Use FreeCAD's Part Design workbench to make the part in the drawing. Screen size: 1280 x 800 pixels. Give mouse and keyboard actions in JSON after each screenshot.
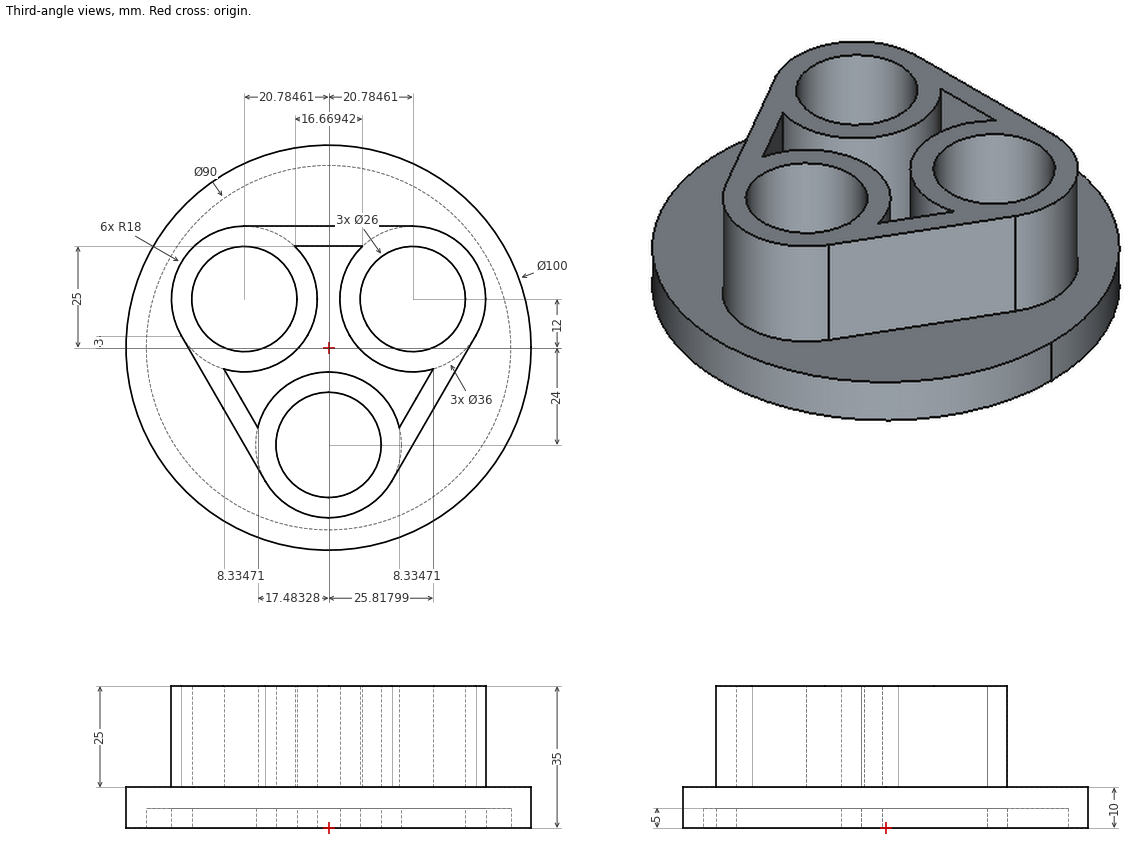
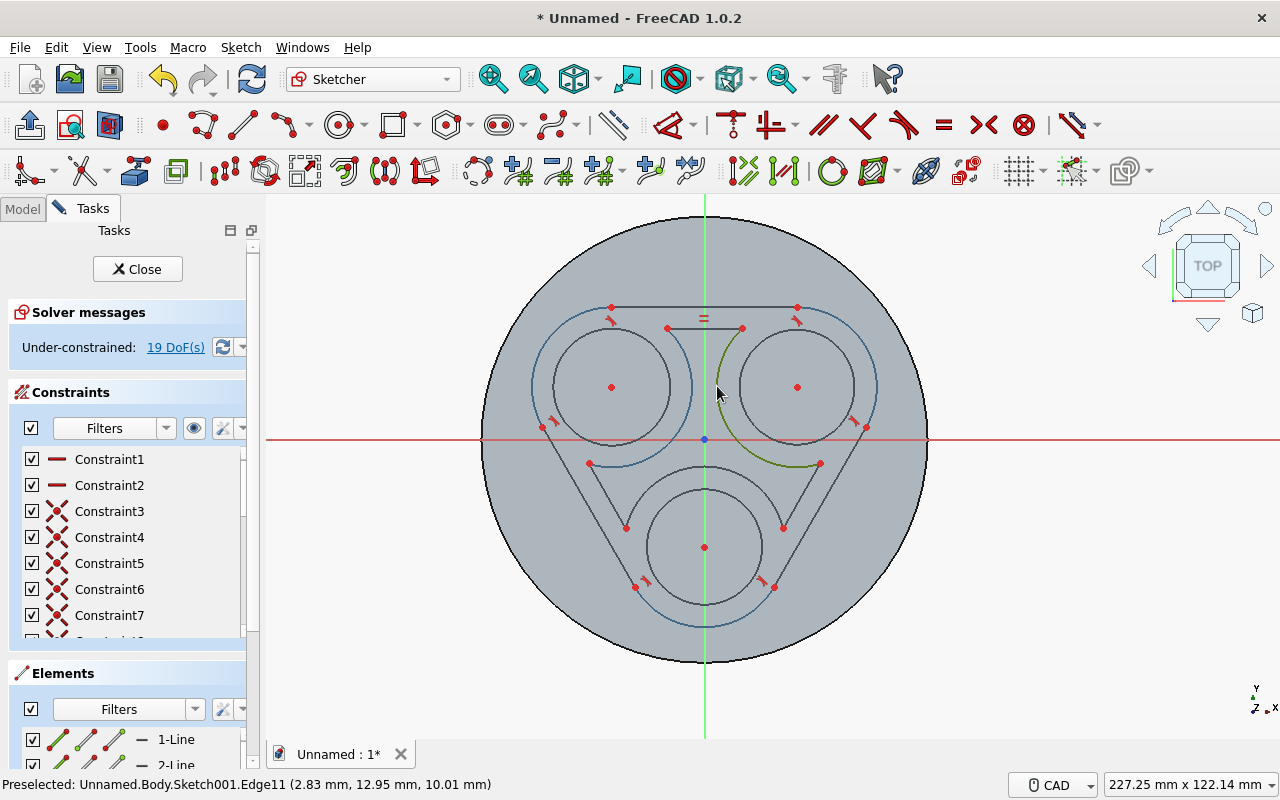
{"action": "left_click", "coordinate": [746, 478]}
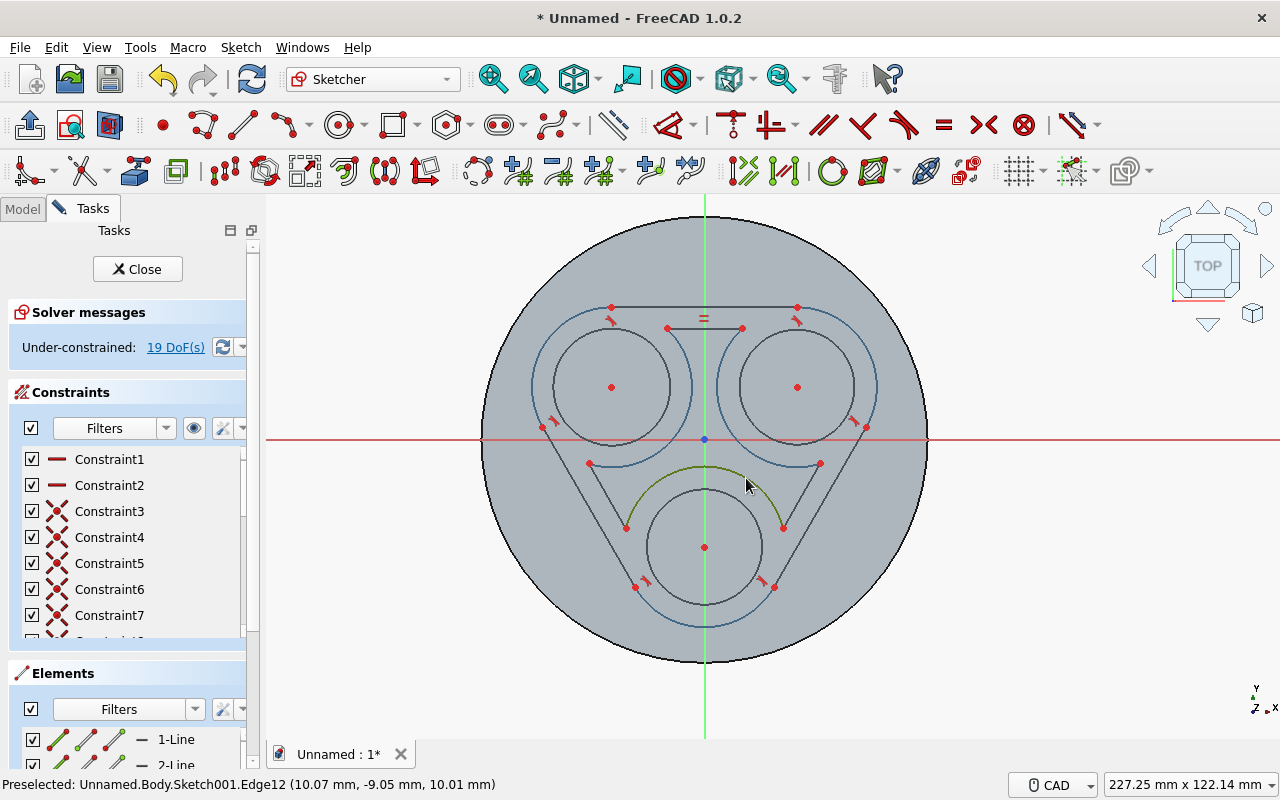
{"action": "left_click", "coordinate": [944, 126]}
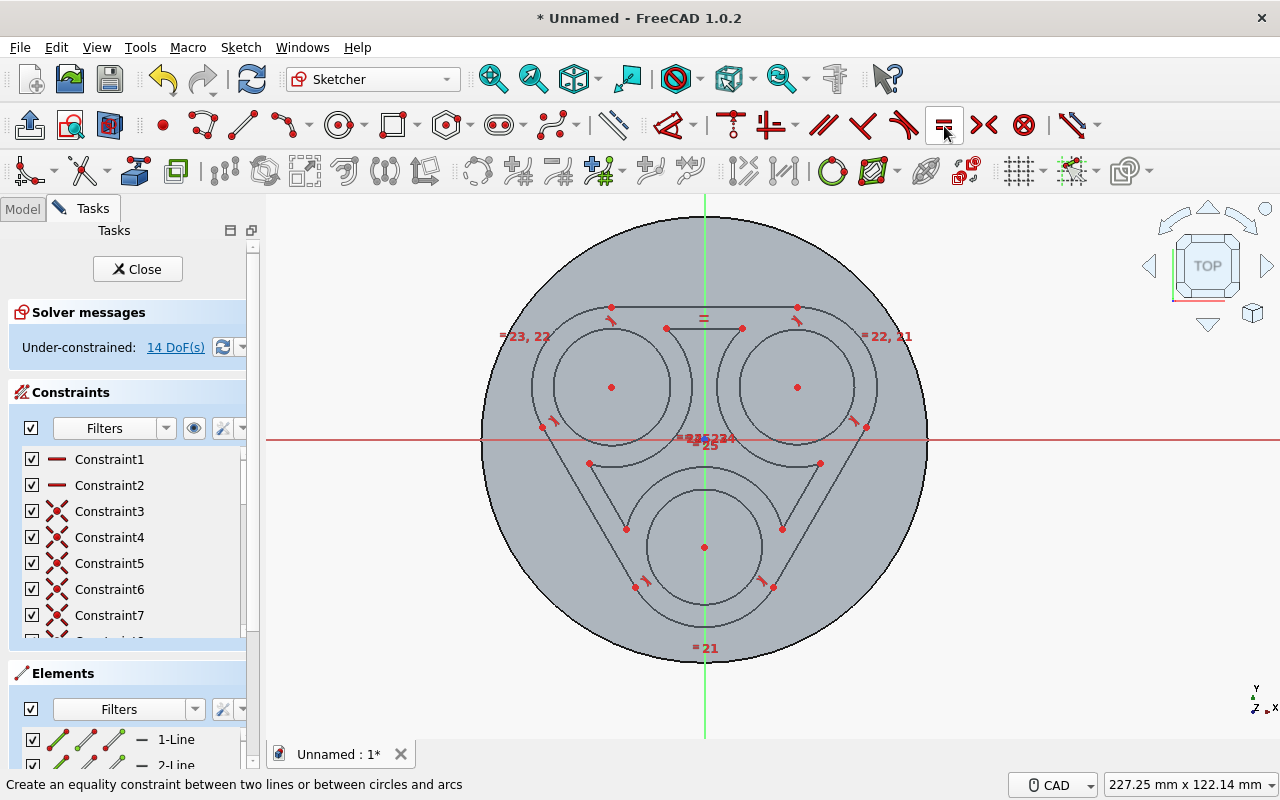
{"action": "left_click", "coordinate": [838, 346]}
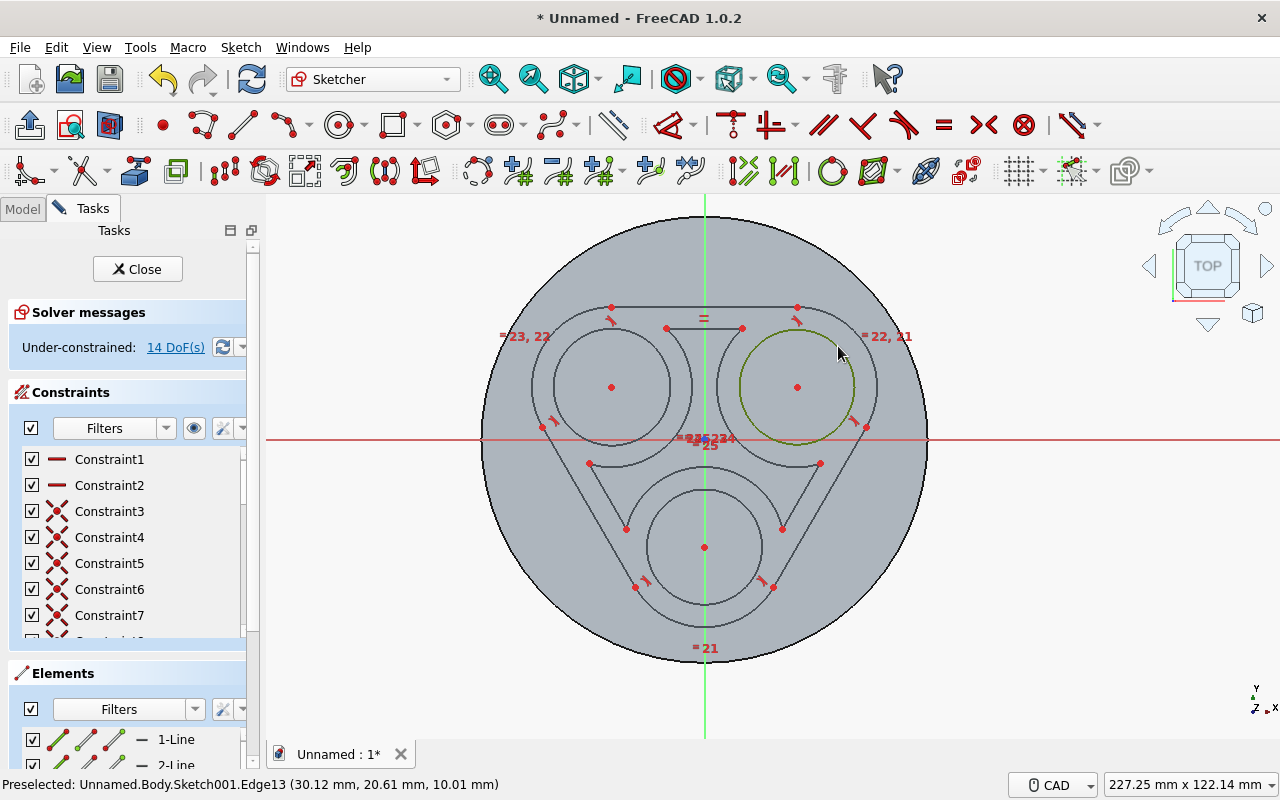
{"action": "left_click", "coordinate": [745, 506]}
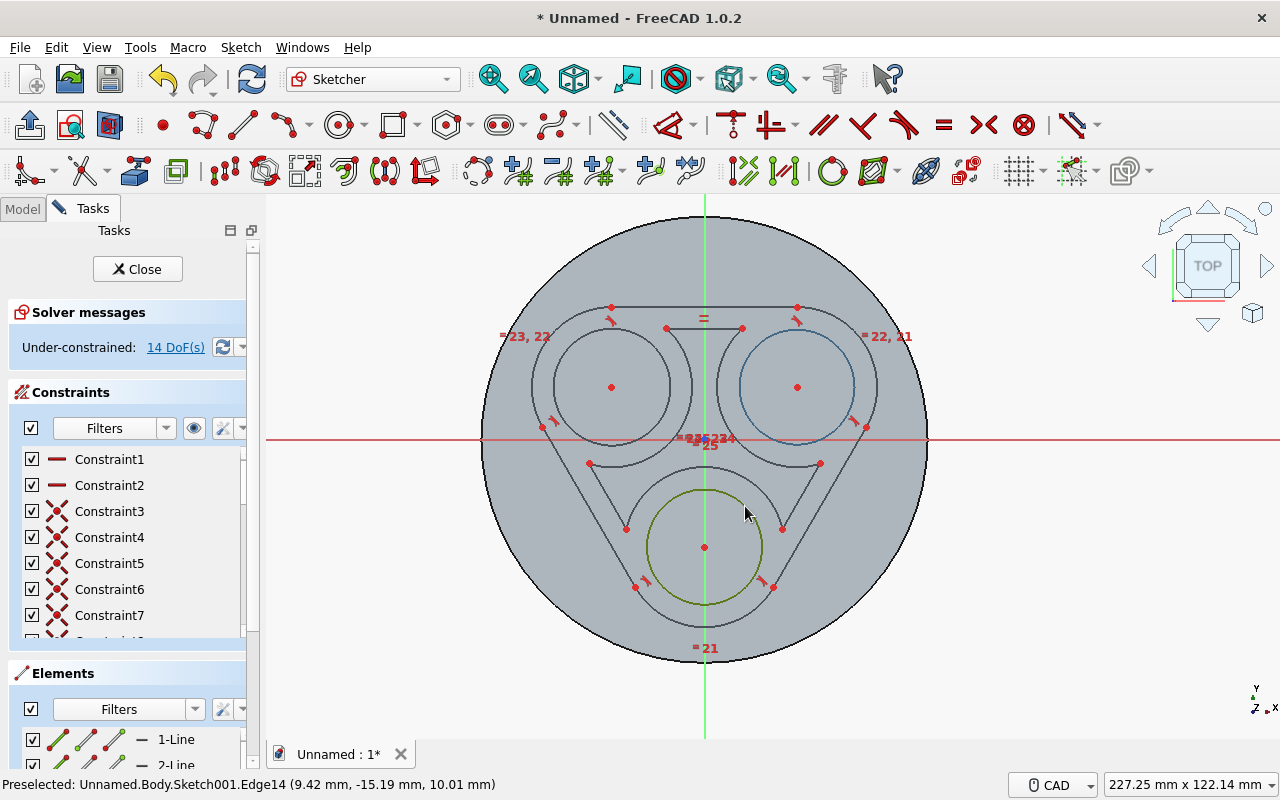
{"action": "left_click", "coordinate": [653, 346]}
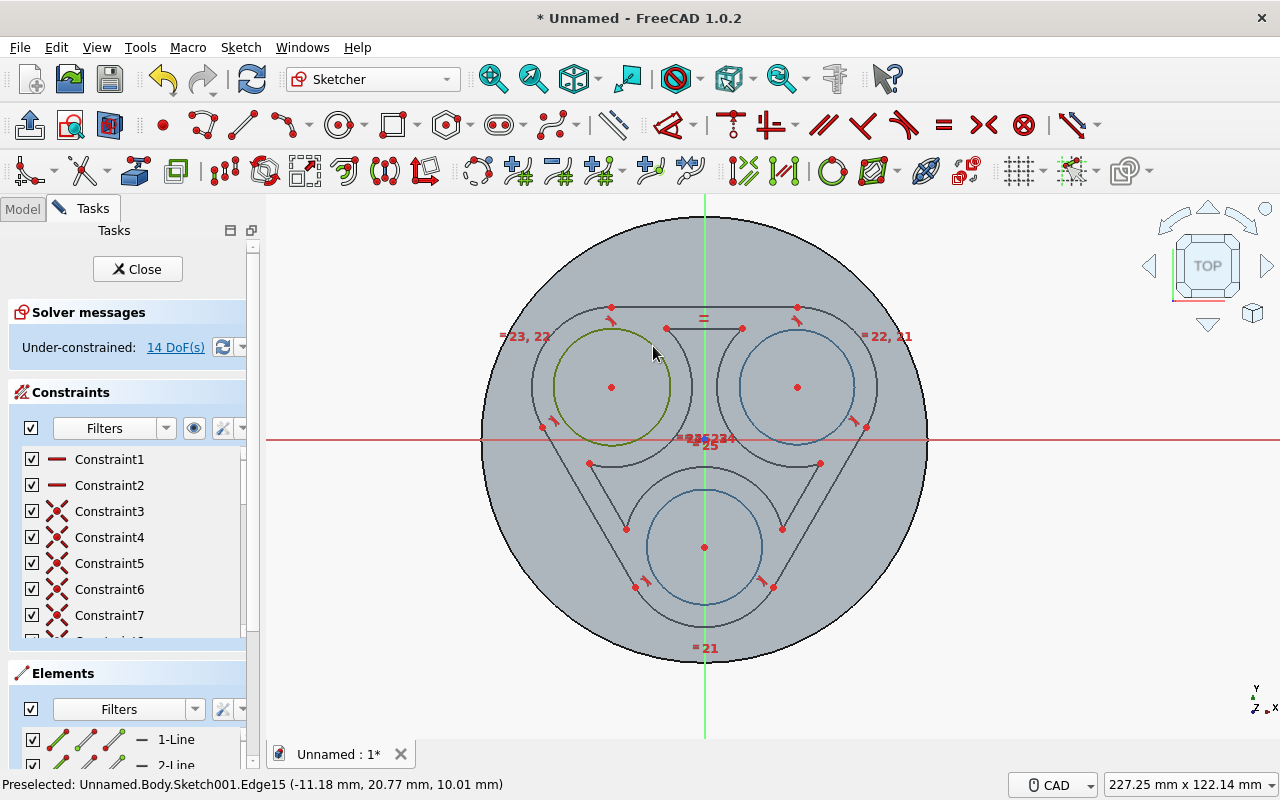
{"action": "left_click", "coordinate": [944, 126]}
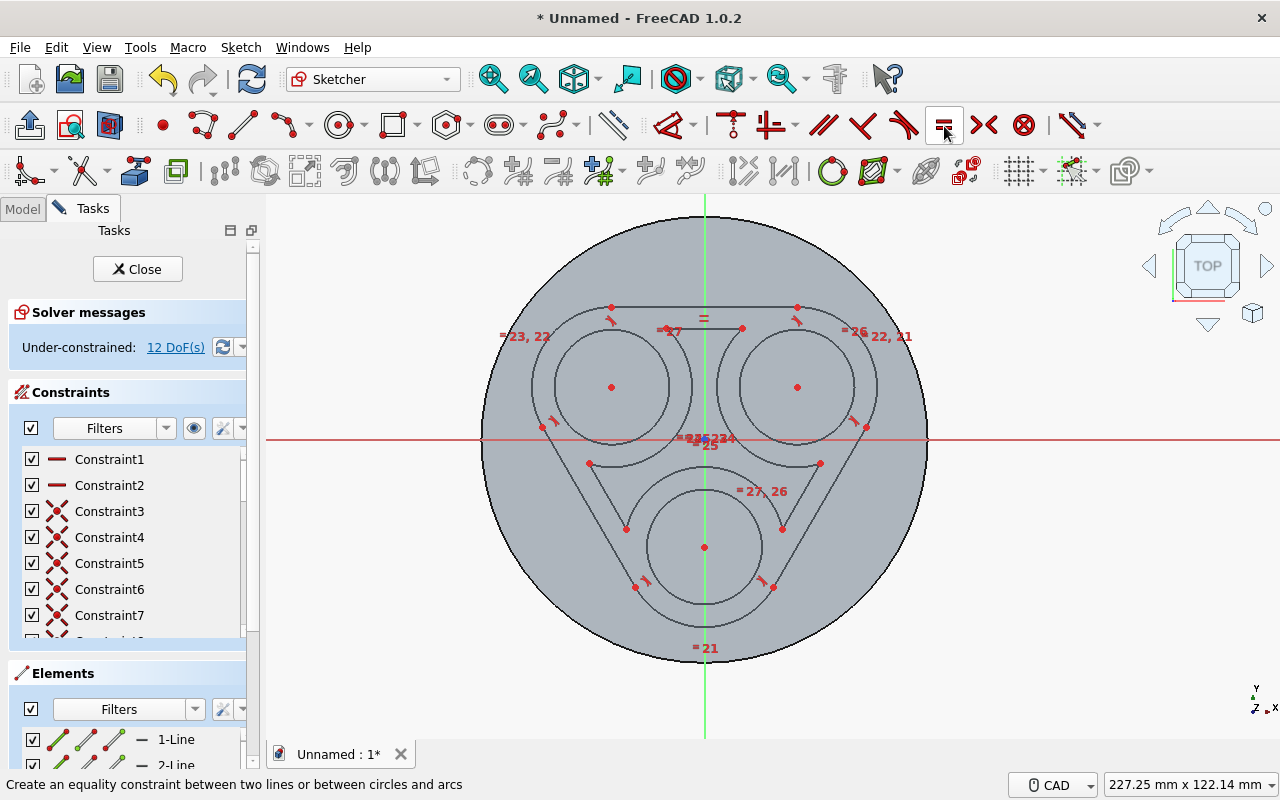
{"action": "left_click", "coordinate": [704, 547]}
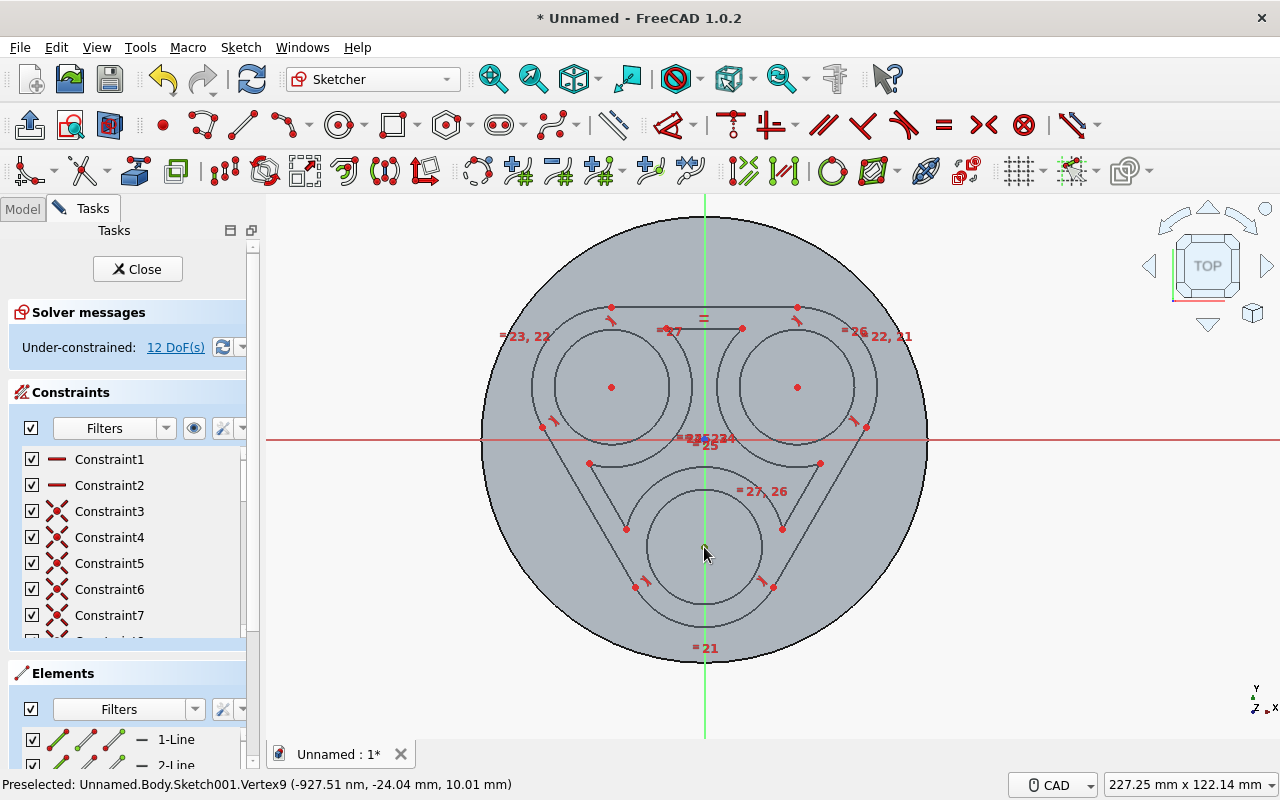
{"action": "left_click", "coordinate": [705, 676]}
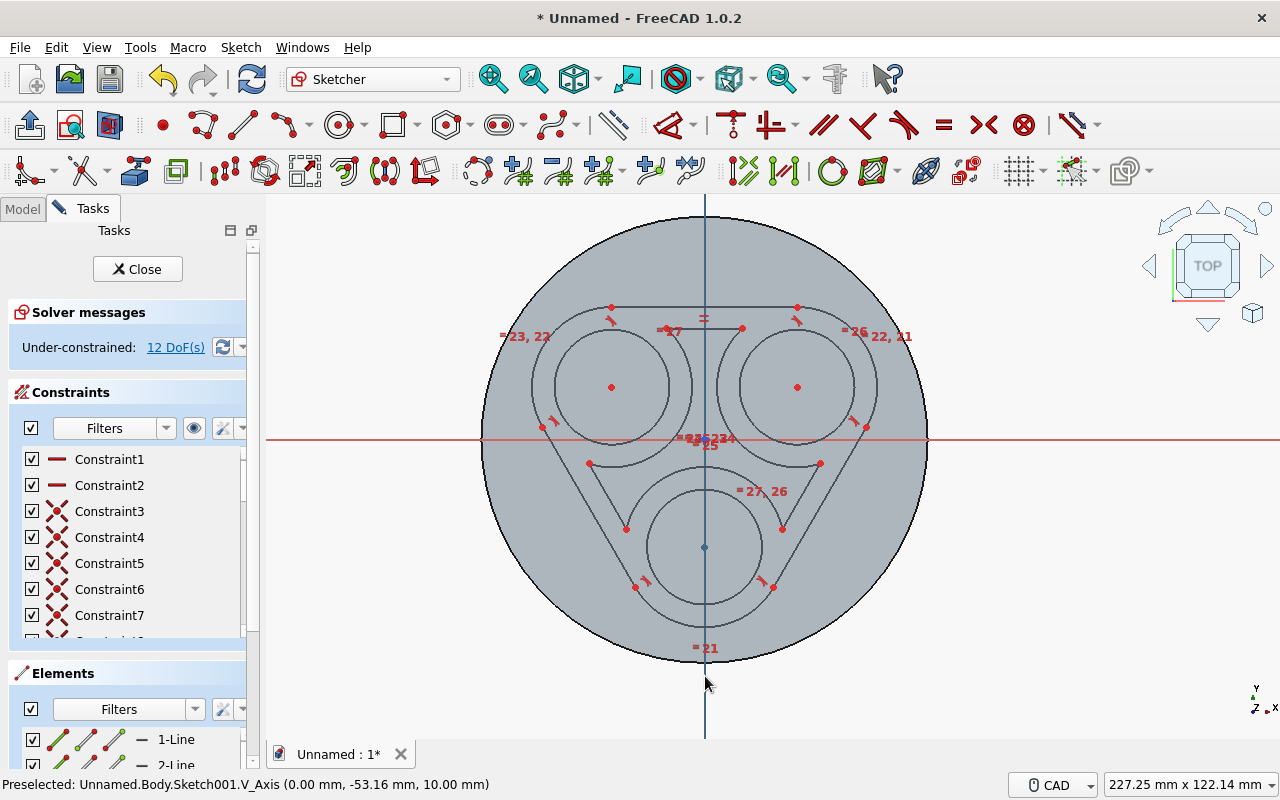
{"action": "left_click", "coordinate": [732, 126]}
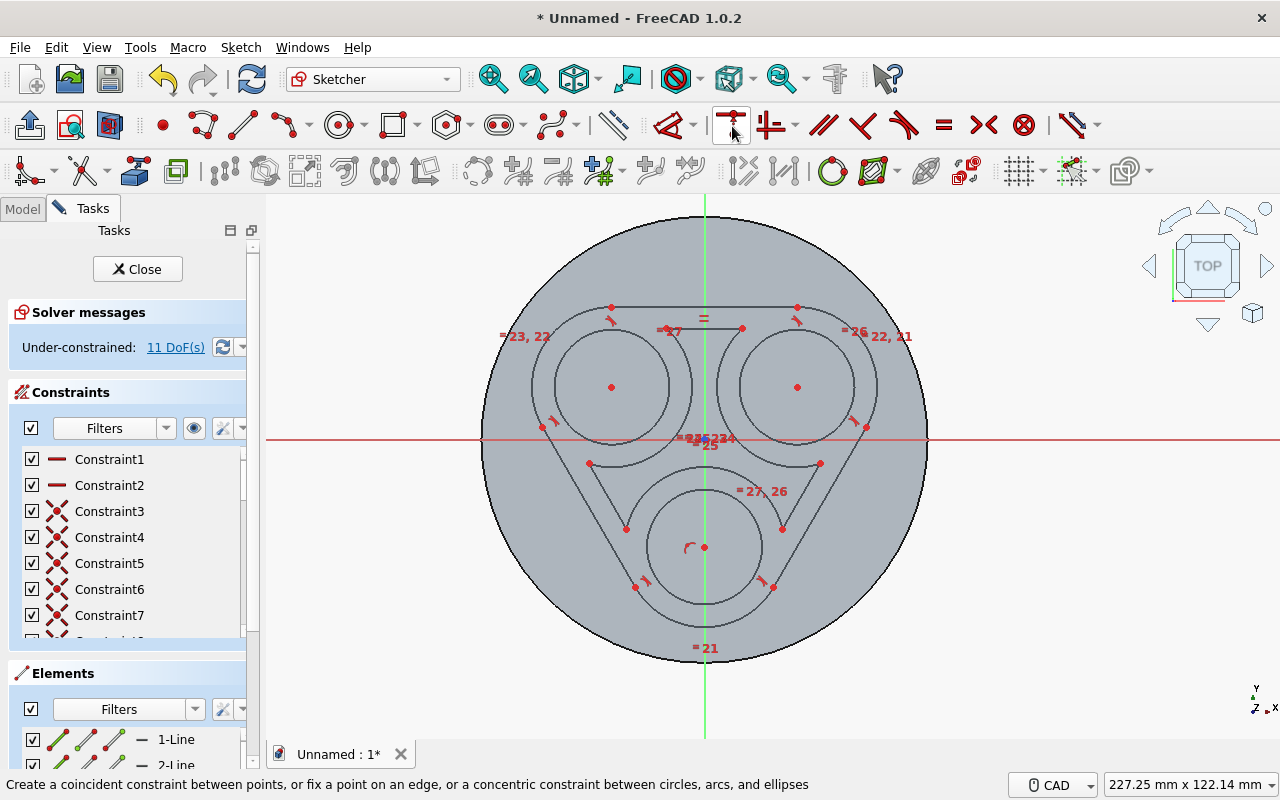
{"action": "left_click", "coordinate": [668, 126]}